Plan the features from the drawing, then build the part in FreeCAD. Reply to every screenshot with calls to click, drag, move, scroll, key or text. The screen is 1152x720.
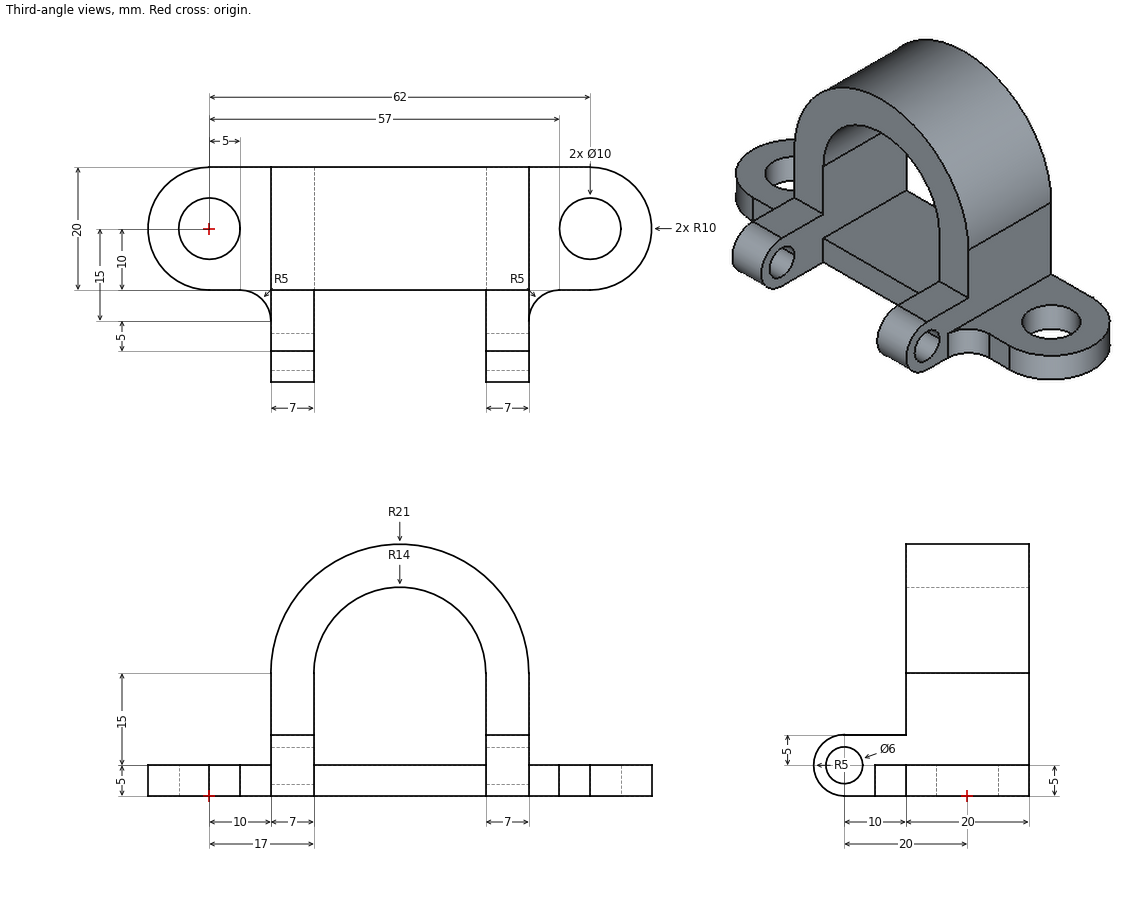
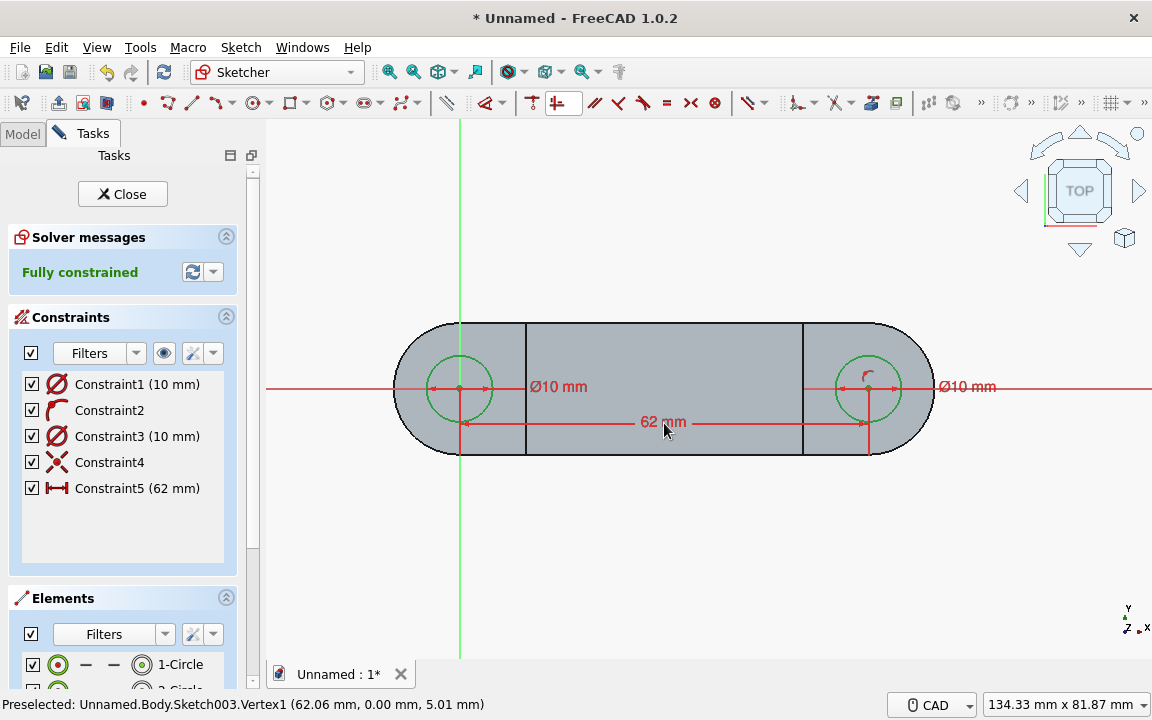
click(123, 194)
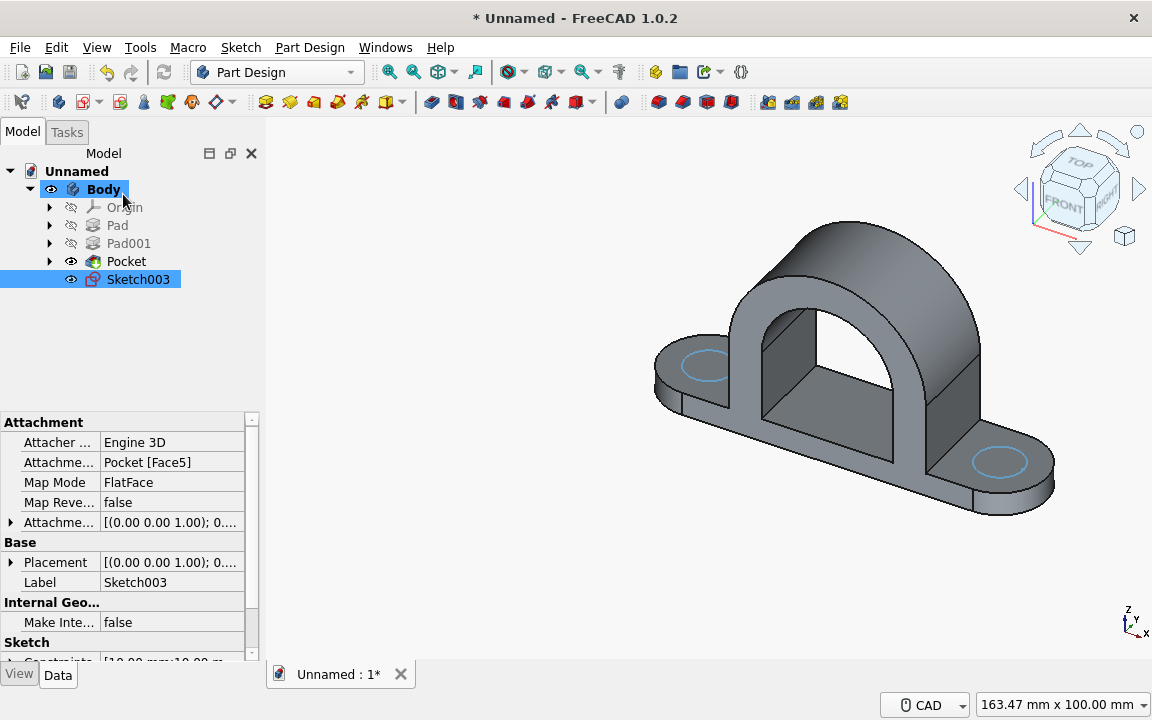
click(432, 102)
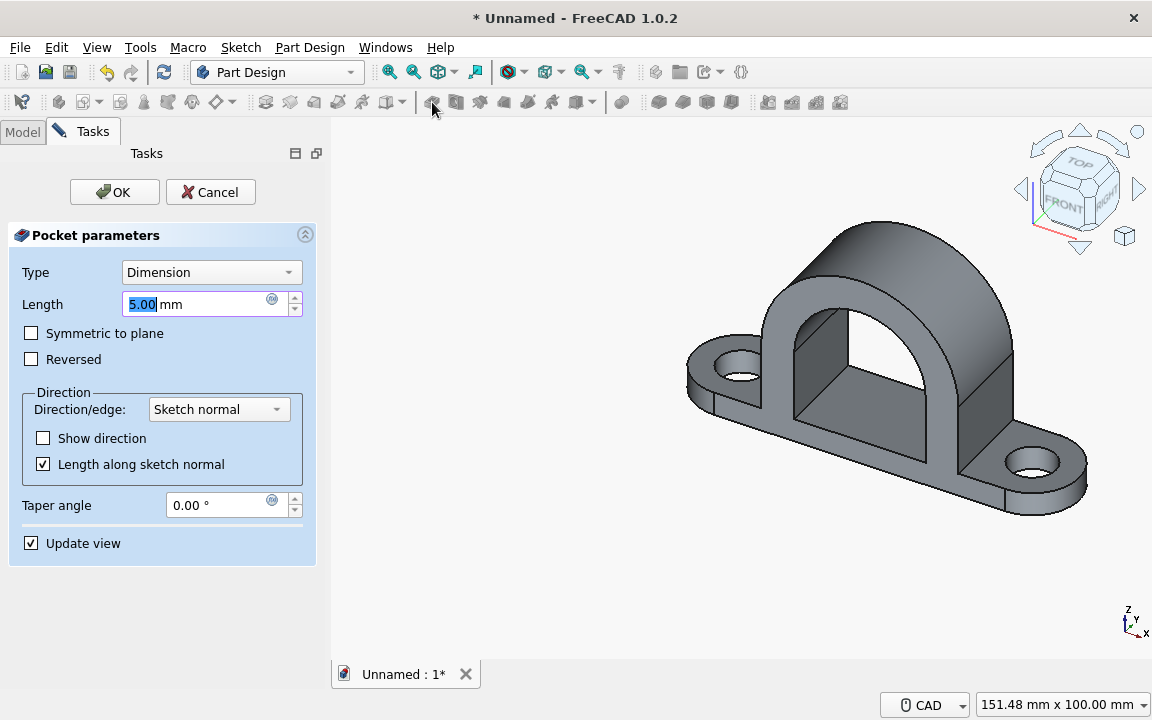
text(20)
key(Tab)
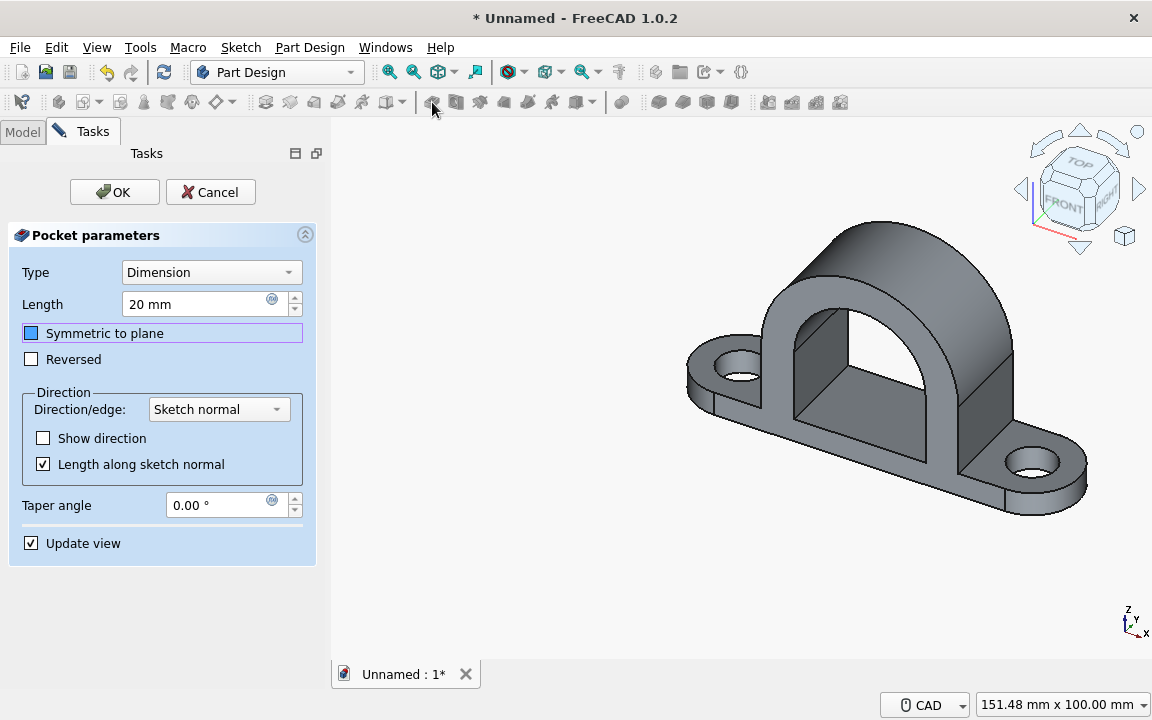
click(115, 192)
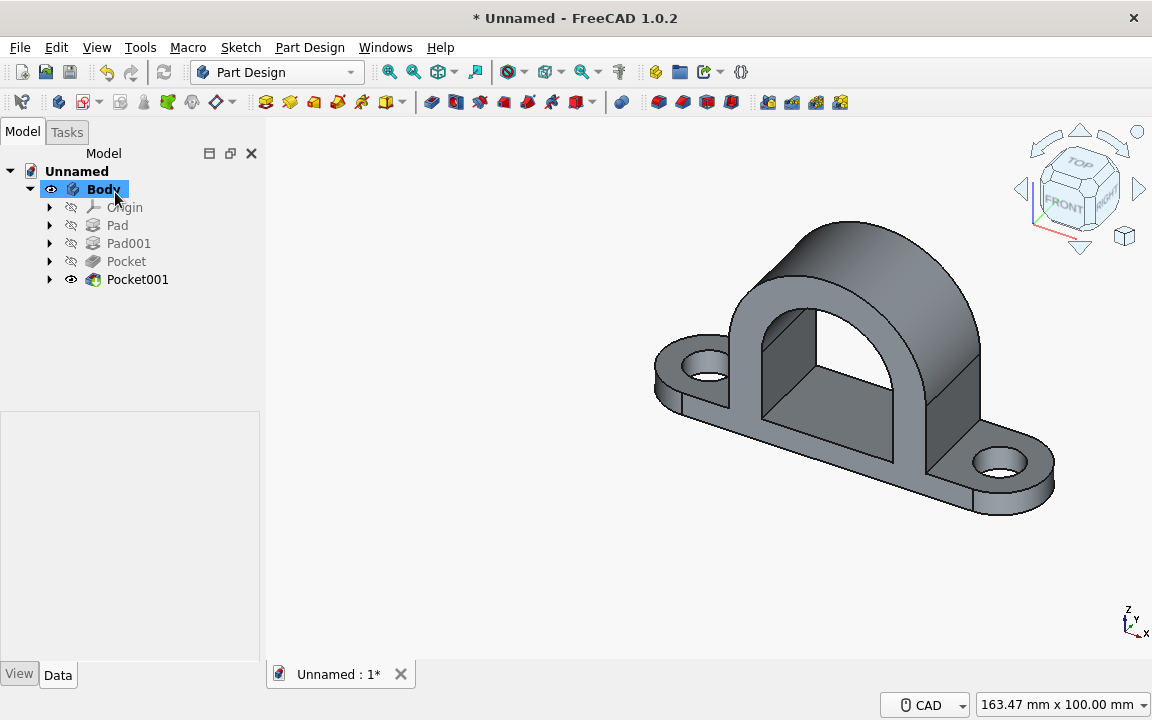
click(720, 389)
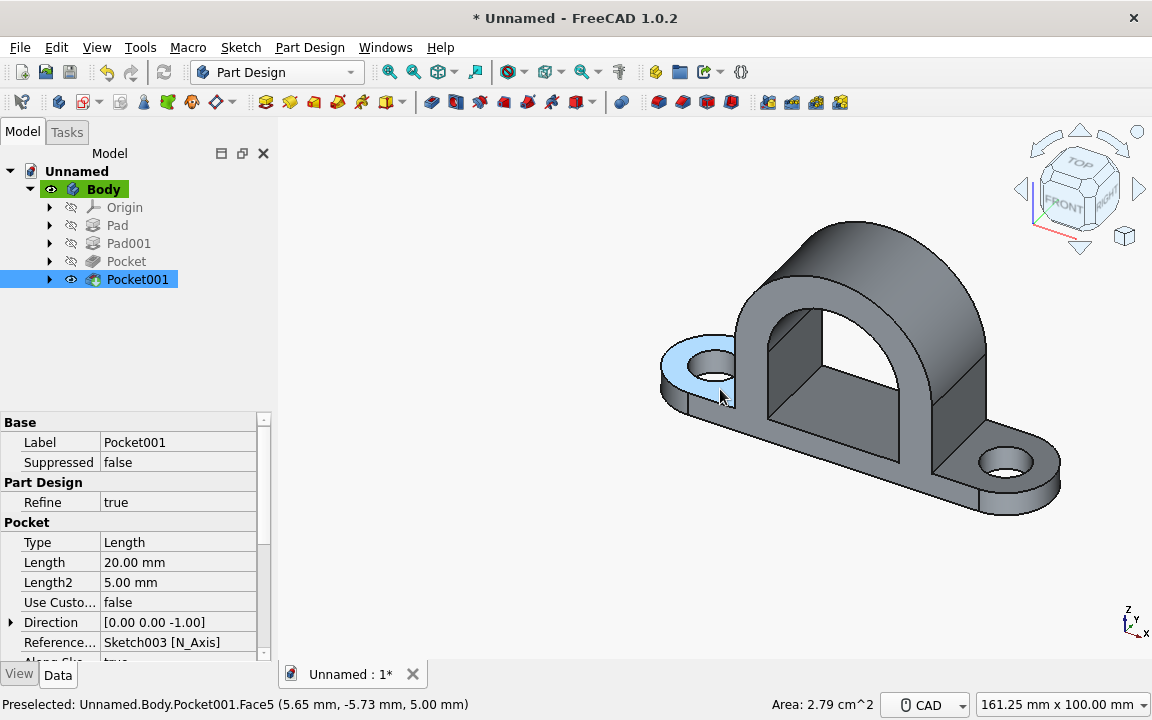
click(84, 102)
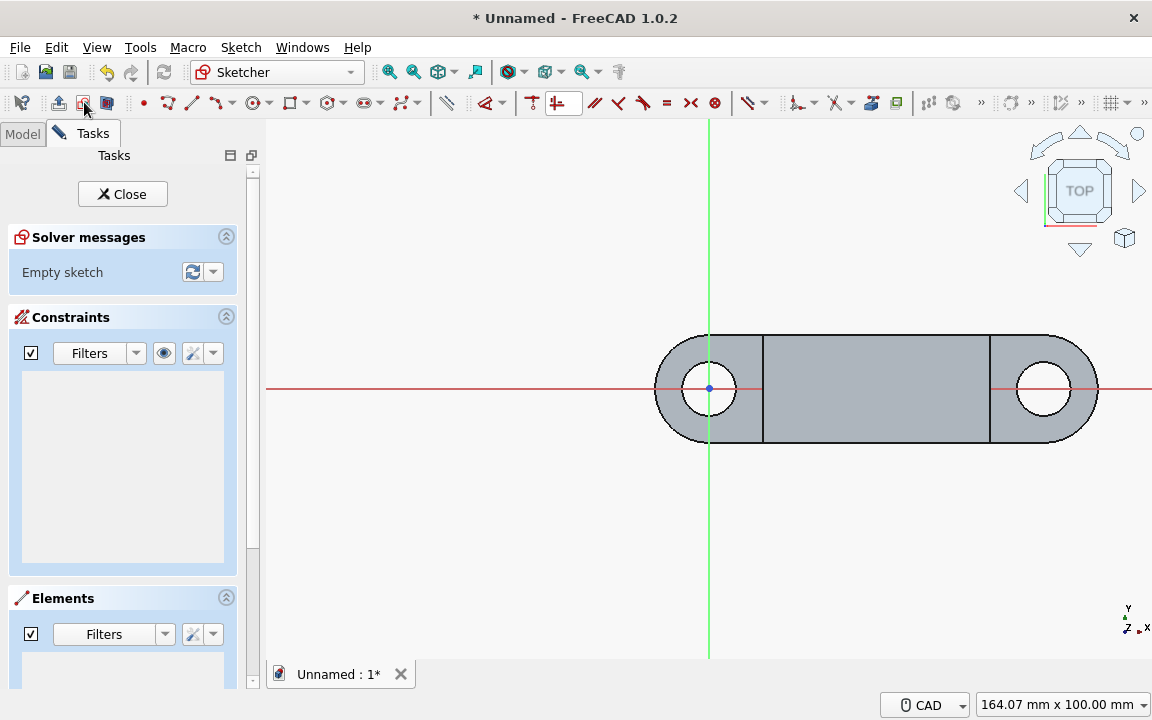
scroll(804, 466, up, 6)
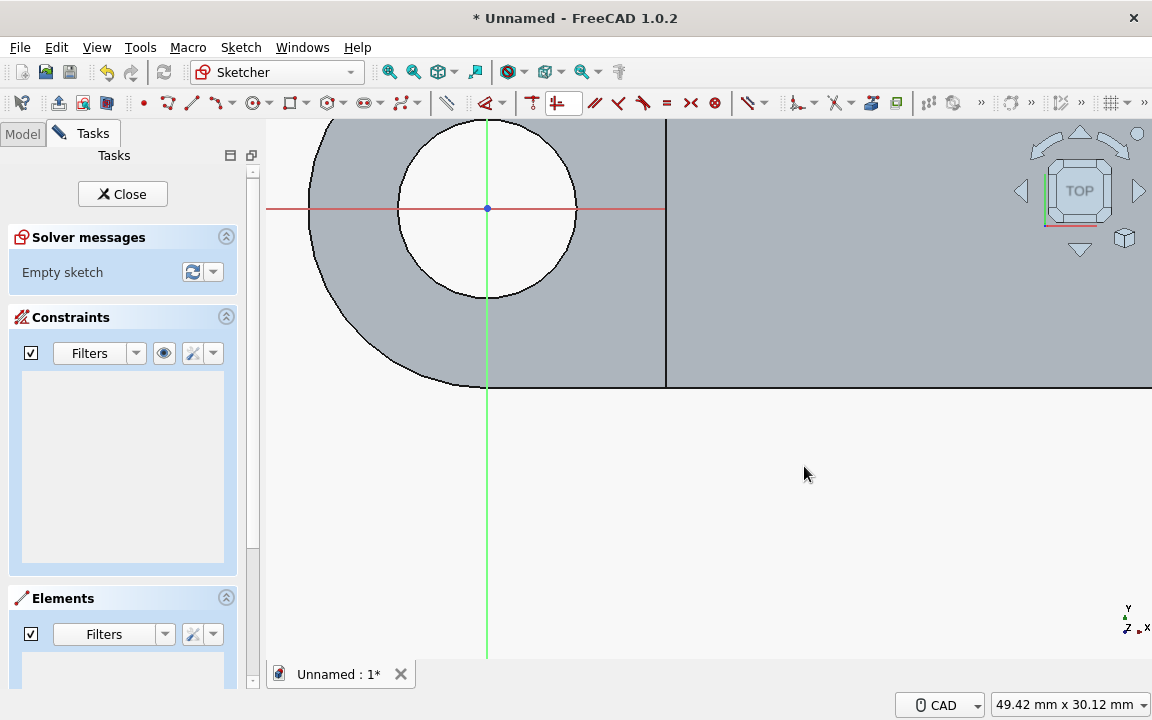
click(168, 104)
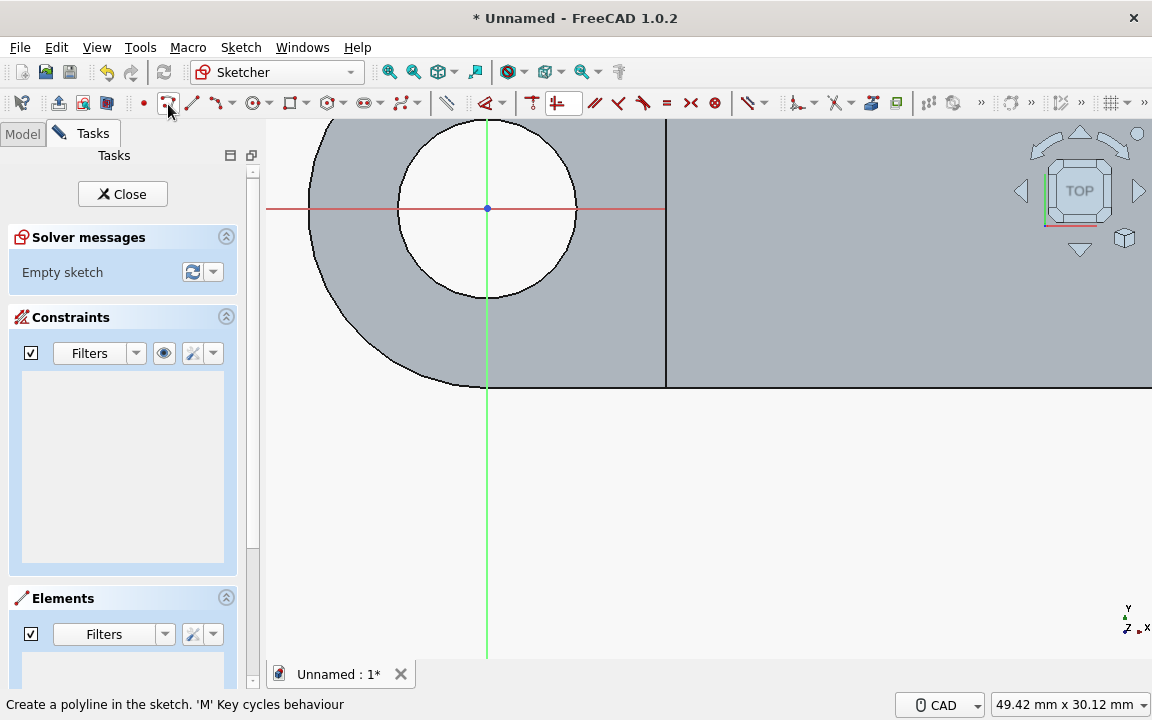
click(666, 478)
click(666, 567)
click(792, 567)
click(792, 388)
click(577, 388)
right_click(577, 388)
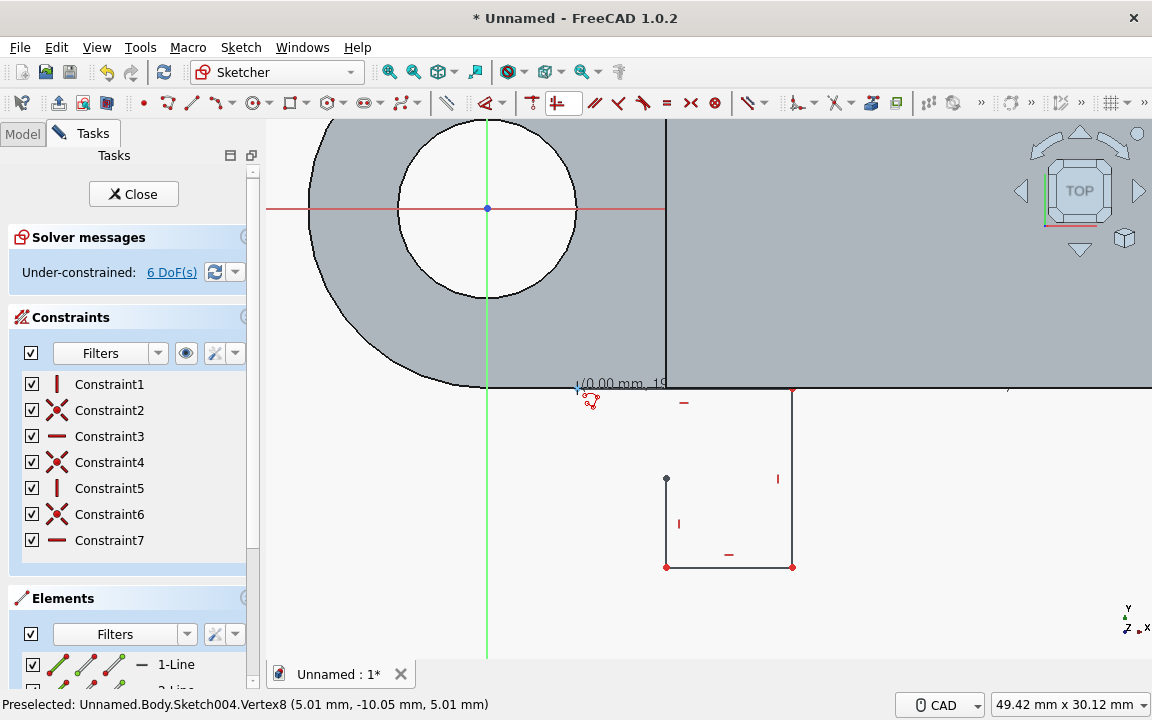
key(g)
key(3)
key(a)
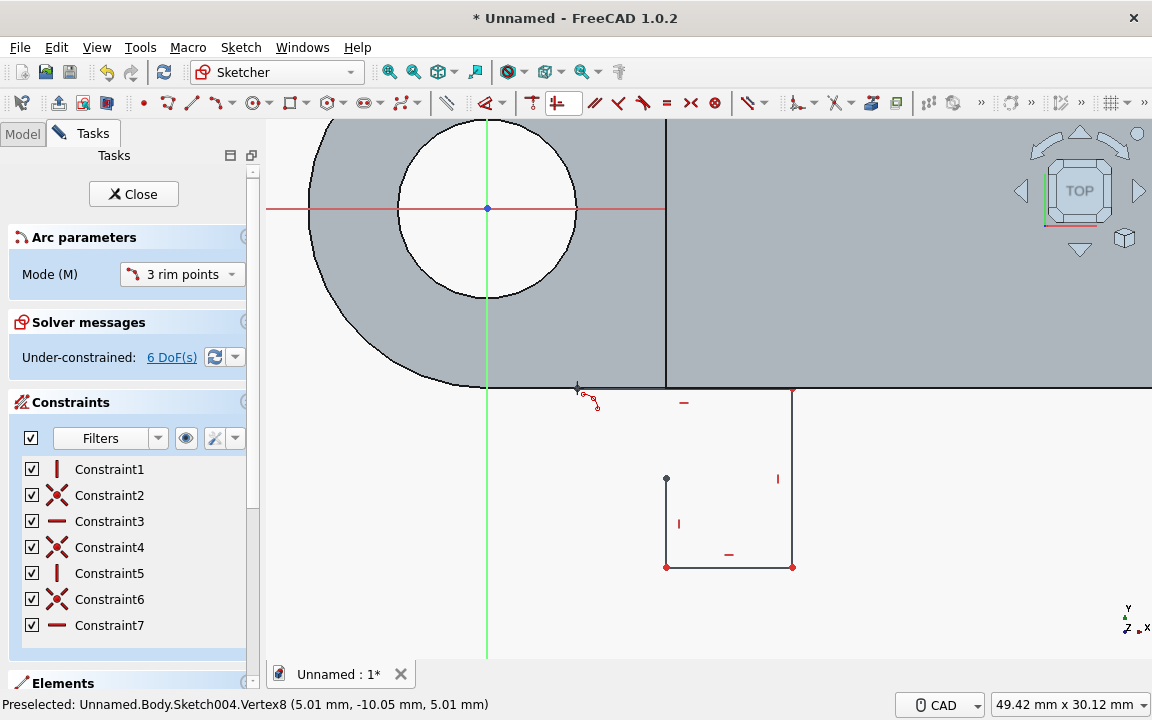
click(577, 389)
click(666, 479)
click(640, 414)
key(Escape)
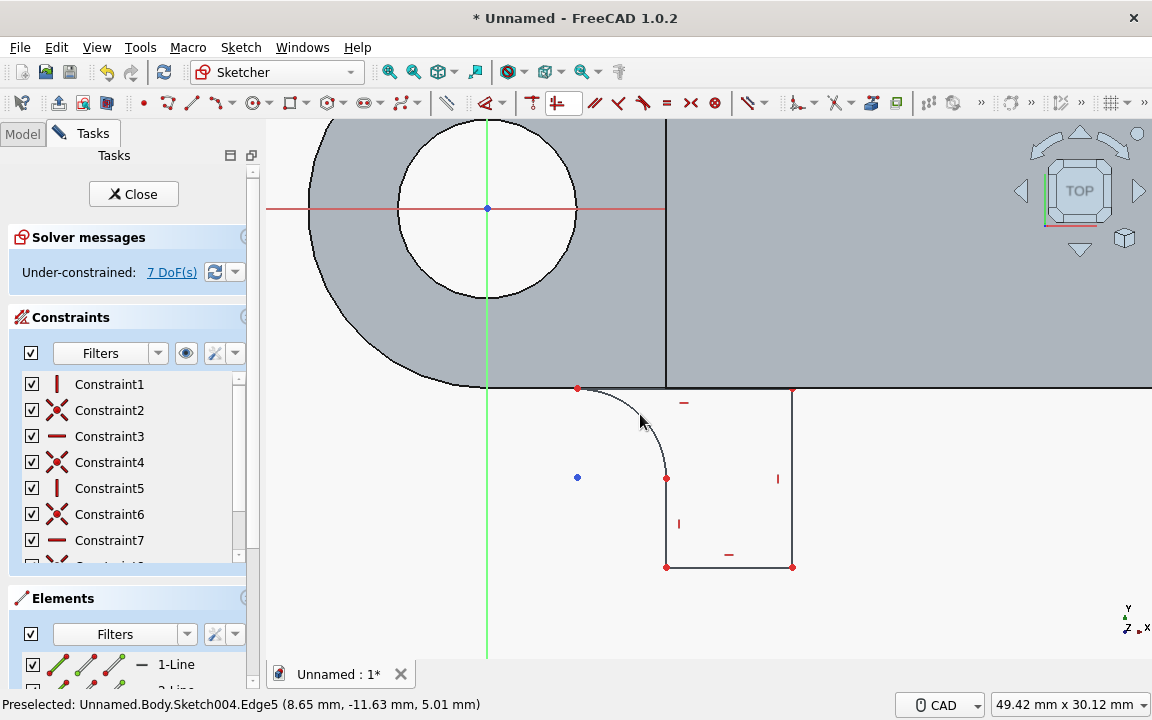
click(666, 506)